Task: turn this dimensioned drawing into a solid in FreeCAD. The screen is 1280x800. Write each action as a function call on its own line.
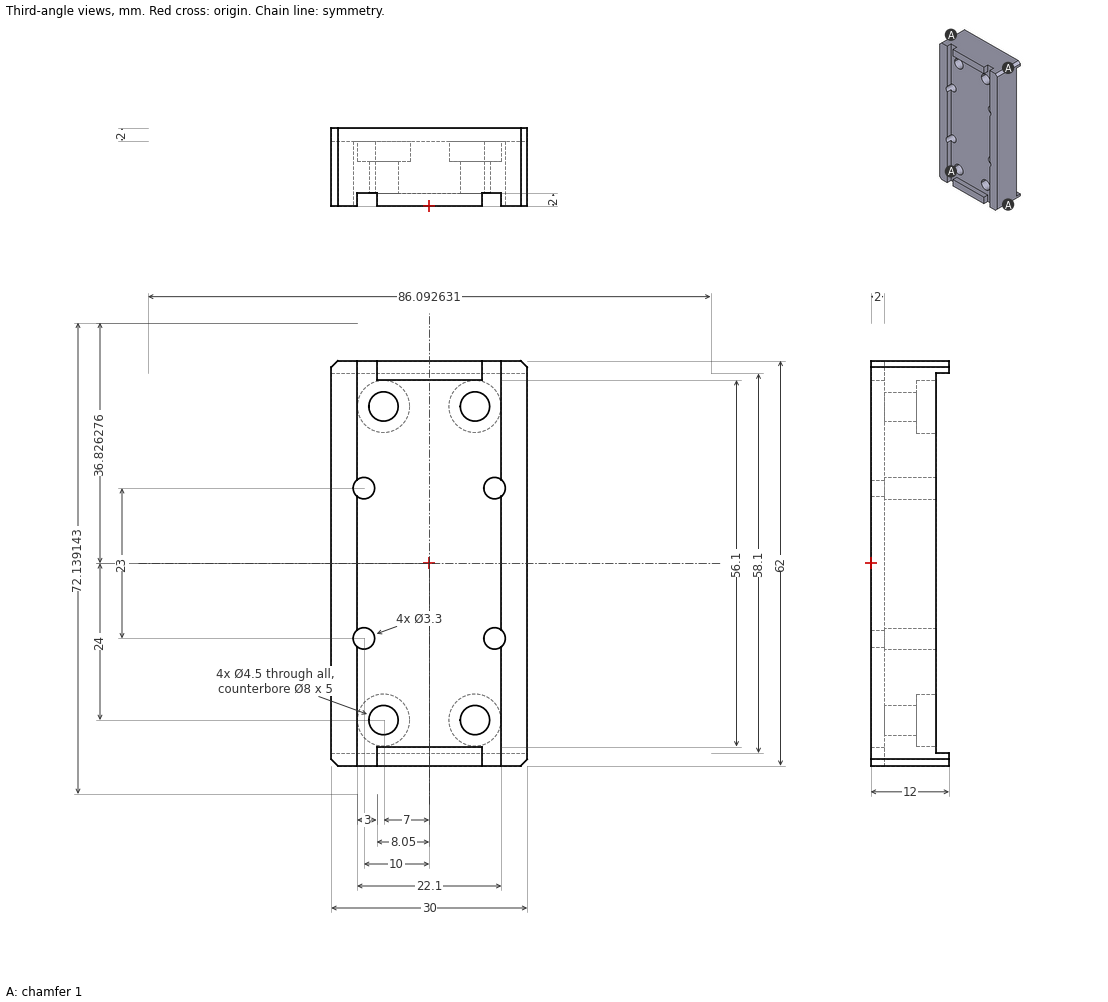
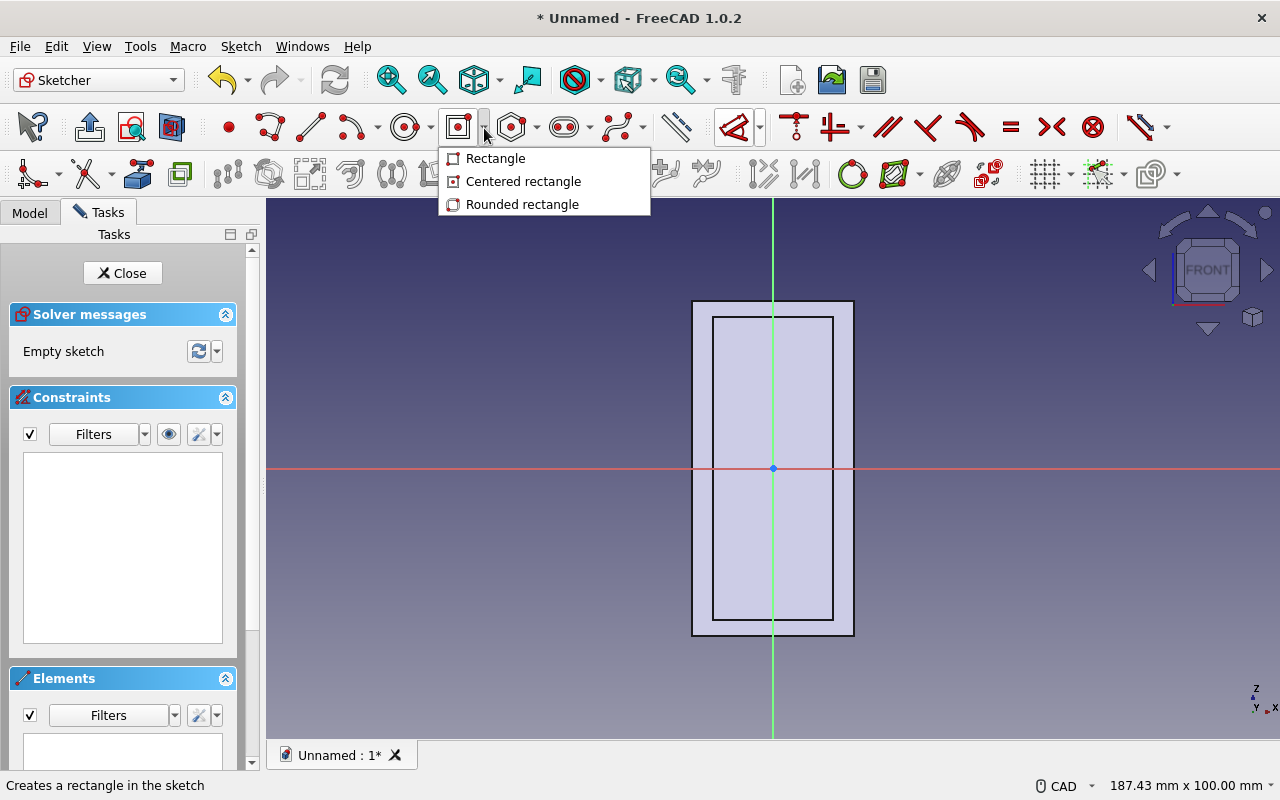
click(544, 158)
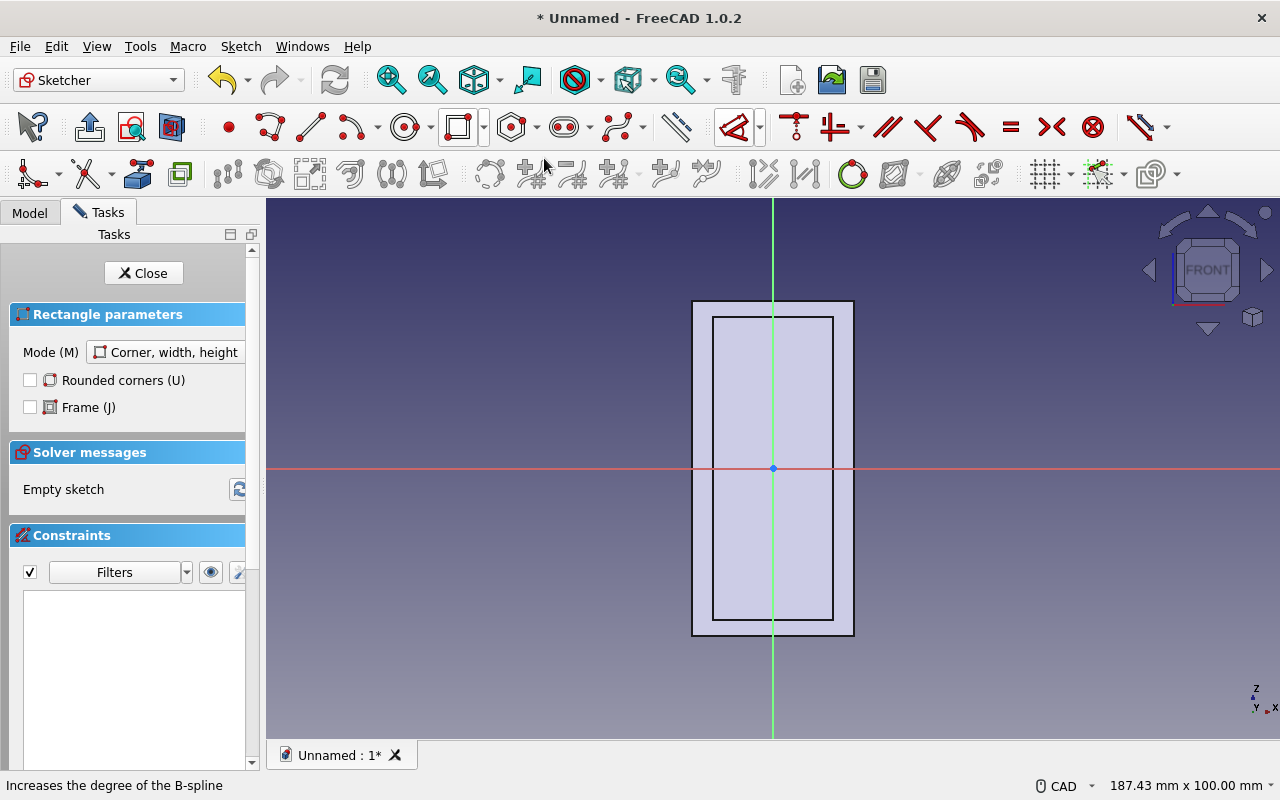
click(713, 269)
click(729, 660)
key(Escape)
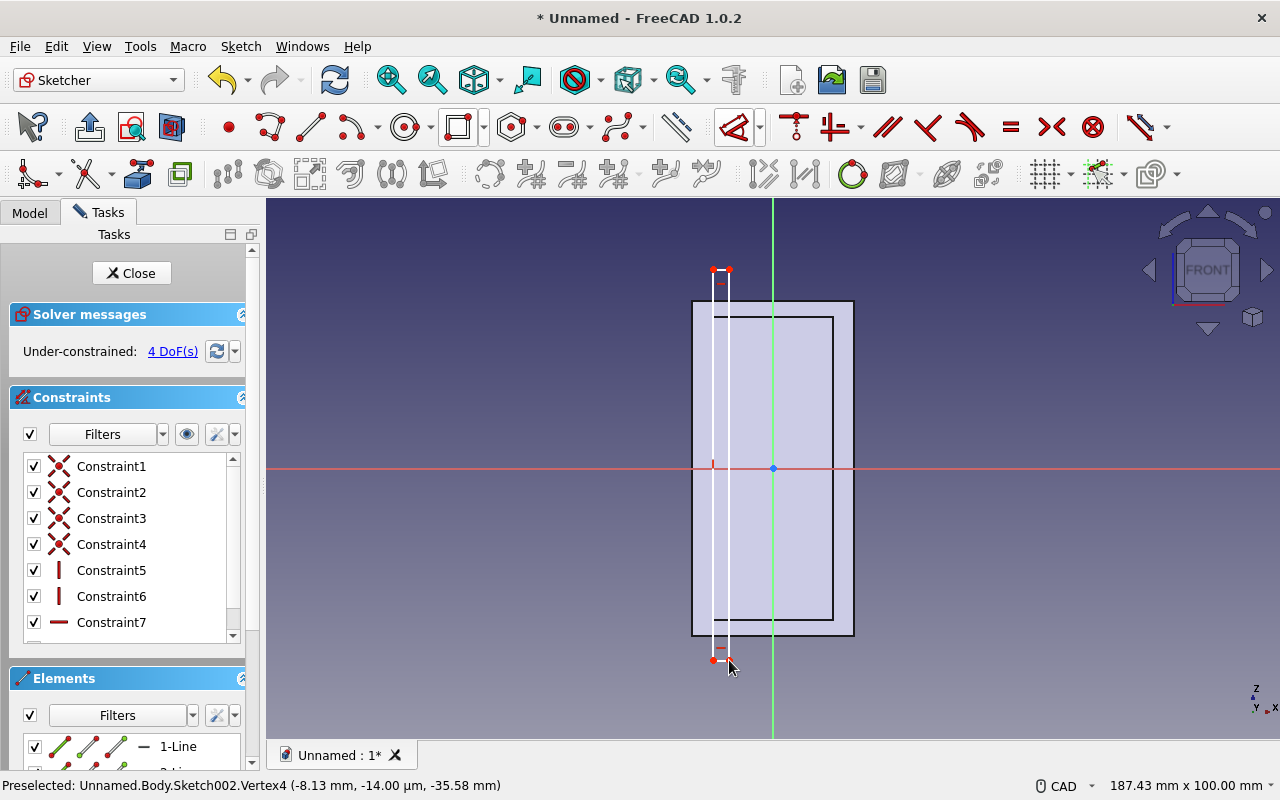
scroll(721, 661, up, 5)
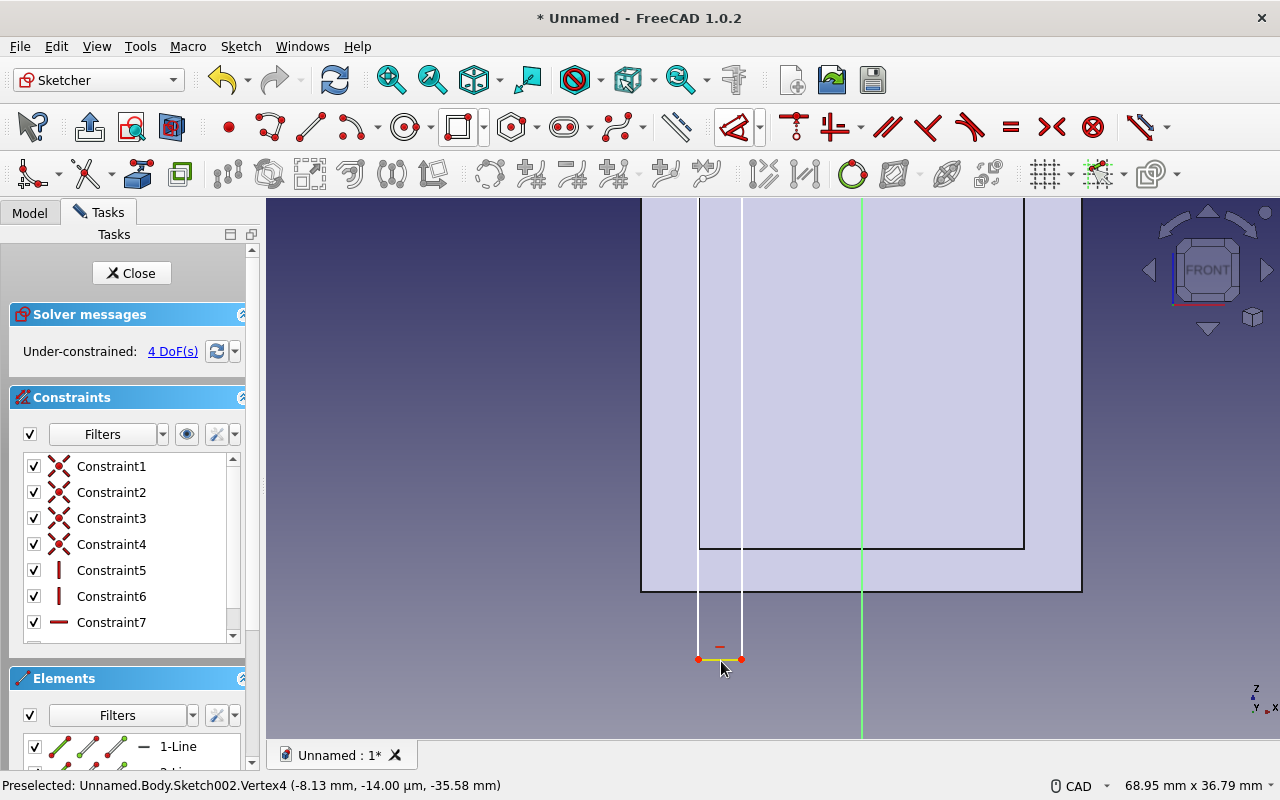
click(720, 660)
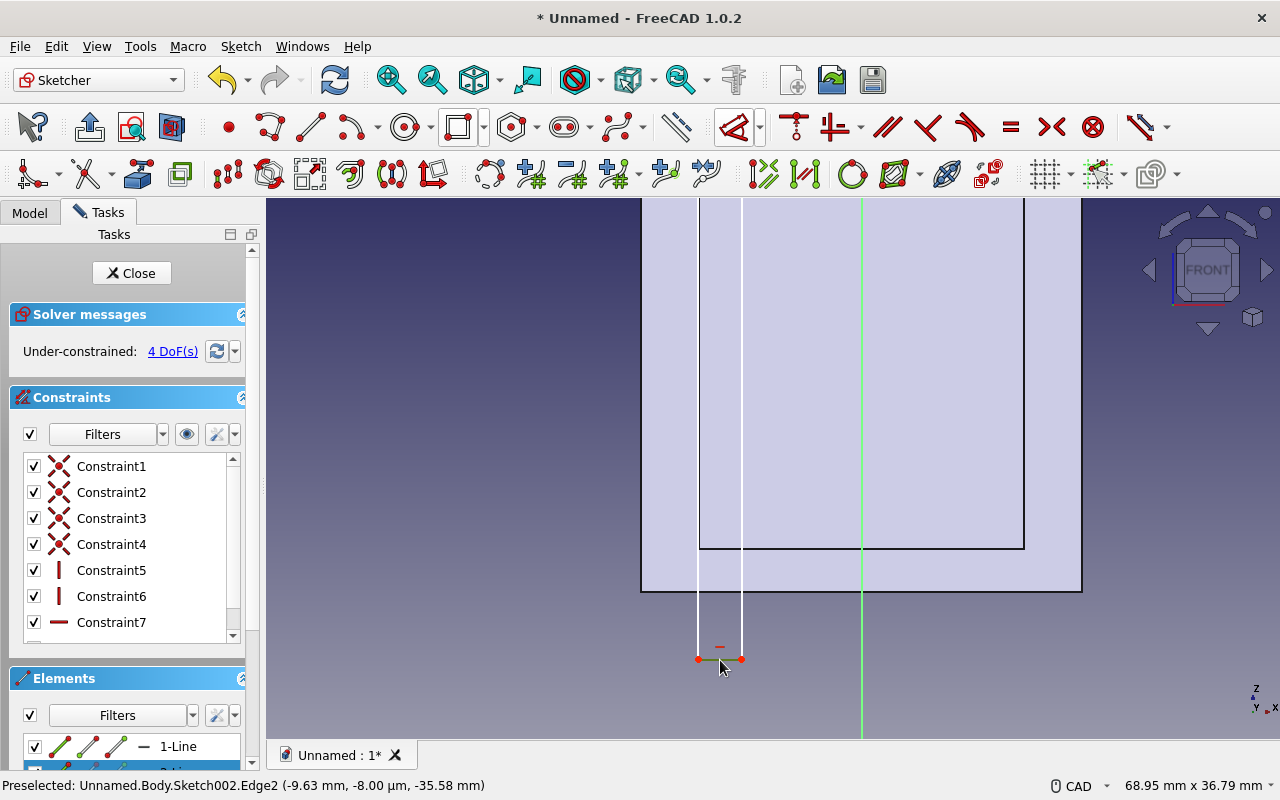
click(760, 128)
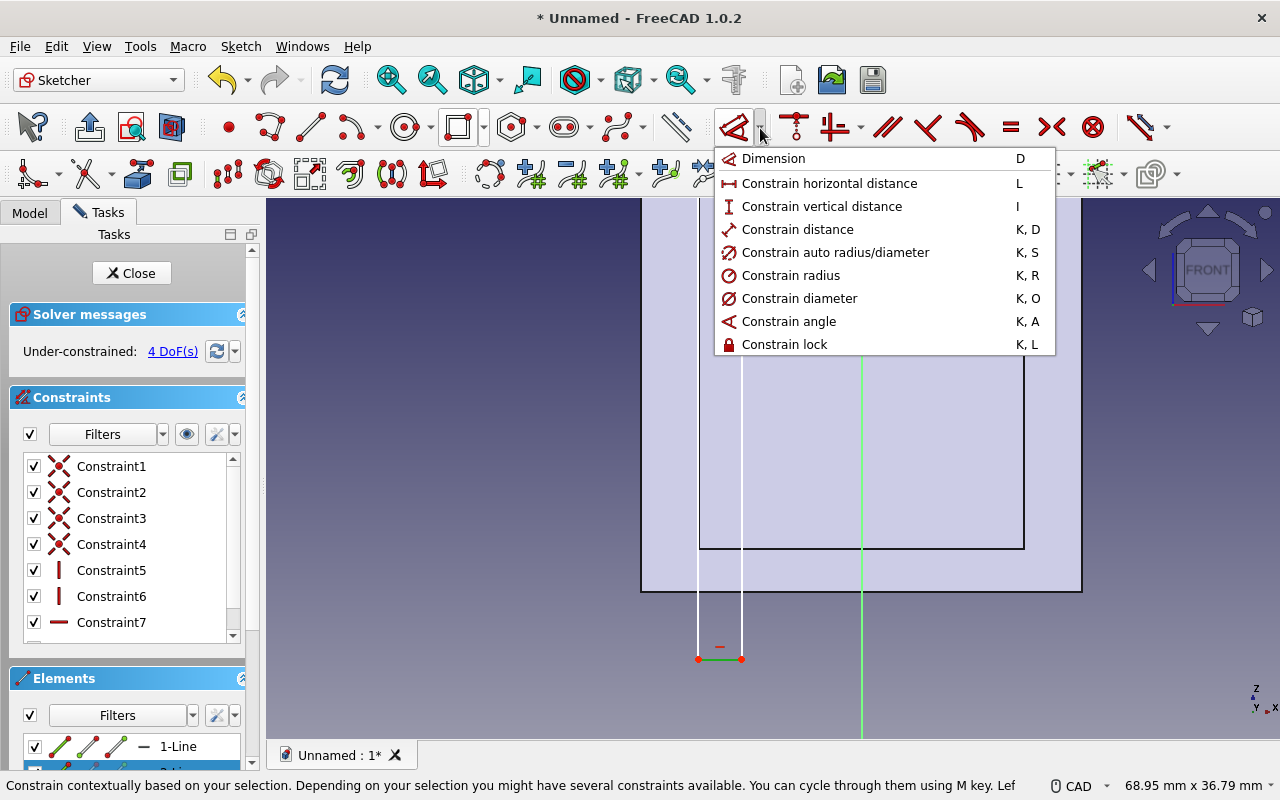
click(885, 184)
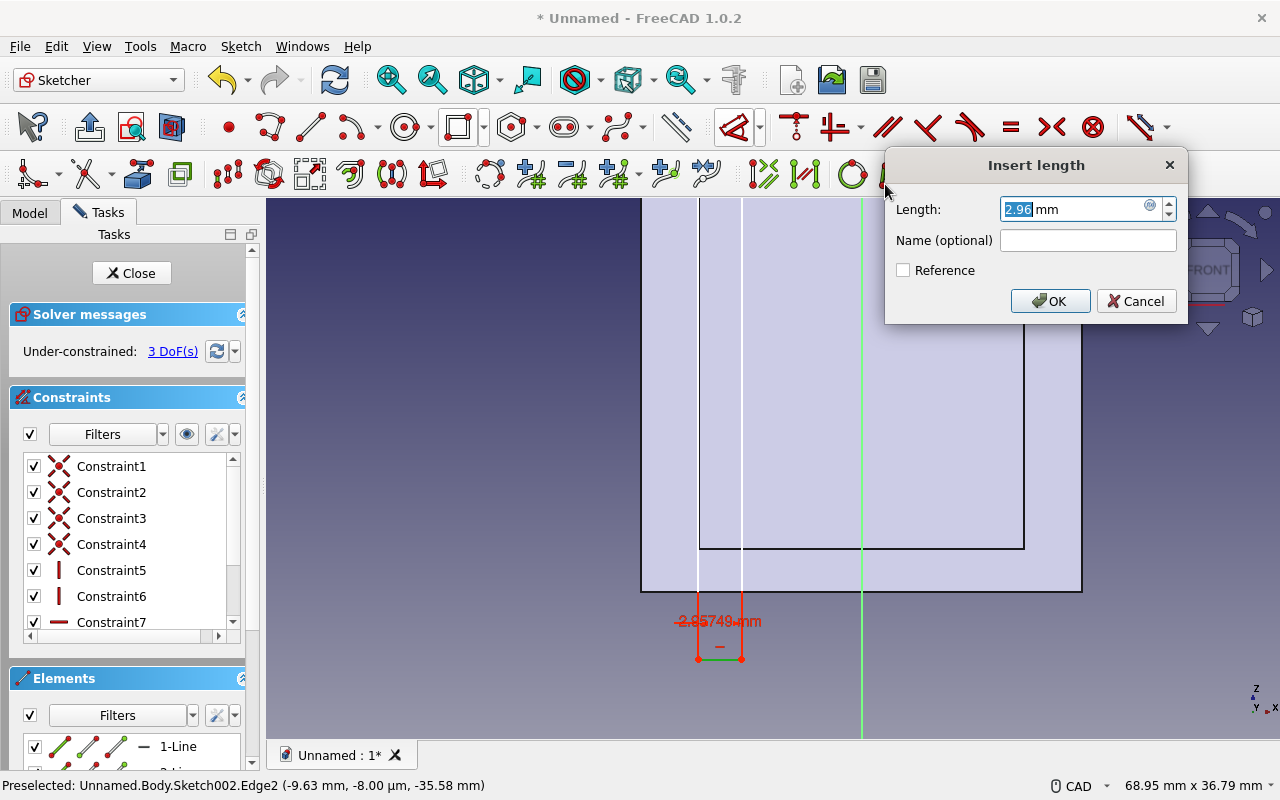
text(3)
key(Return)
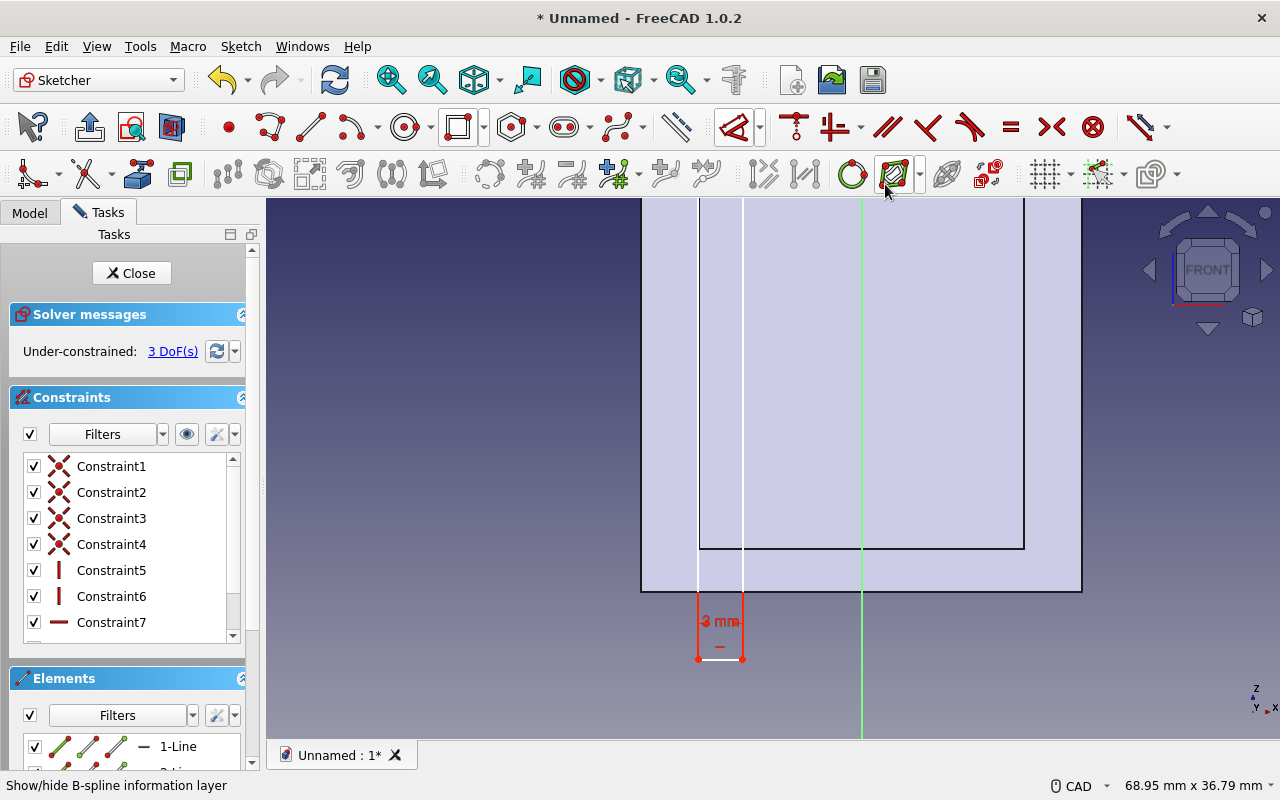
click(743, 660)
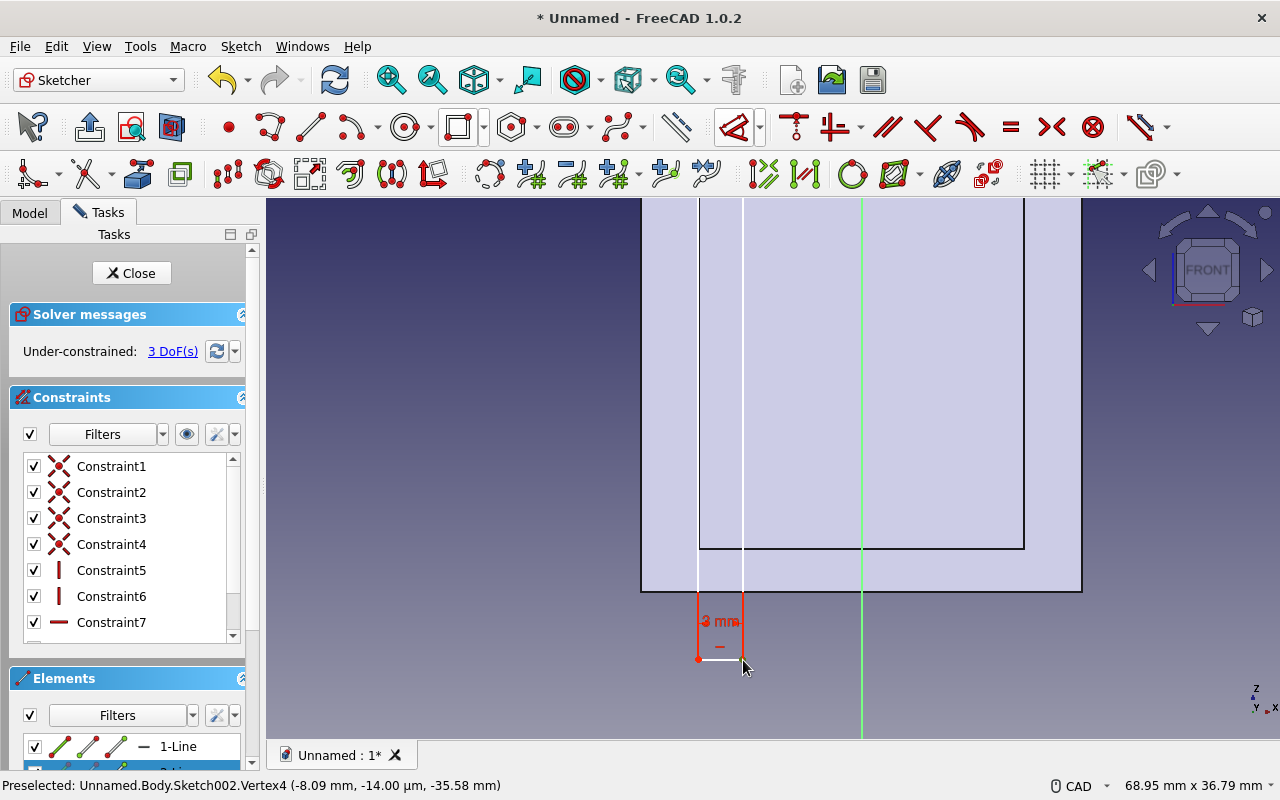
click(760, 128)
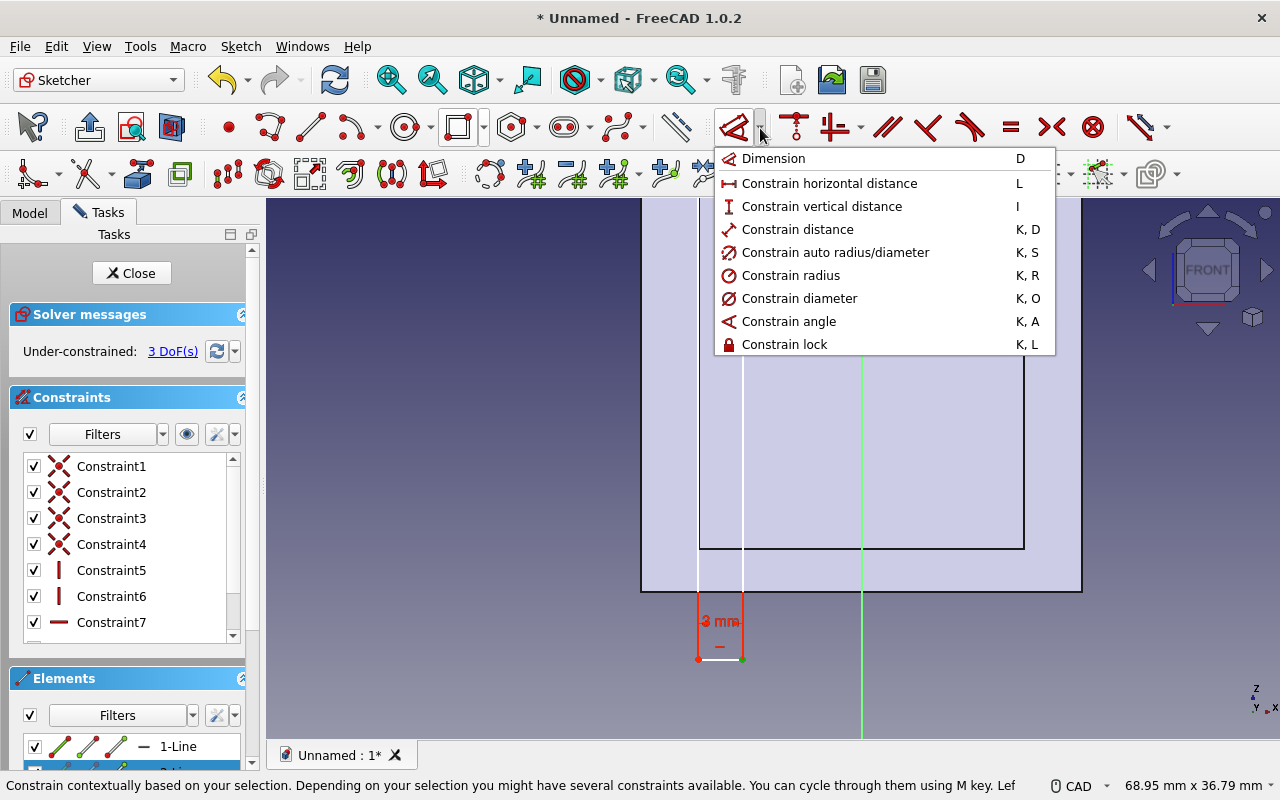
click(885, 184)